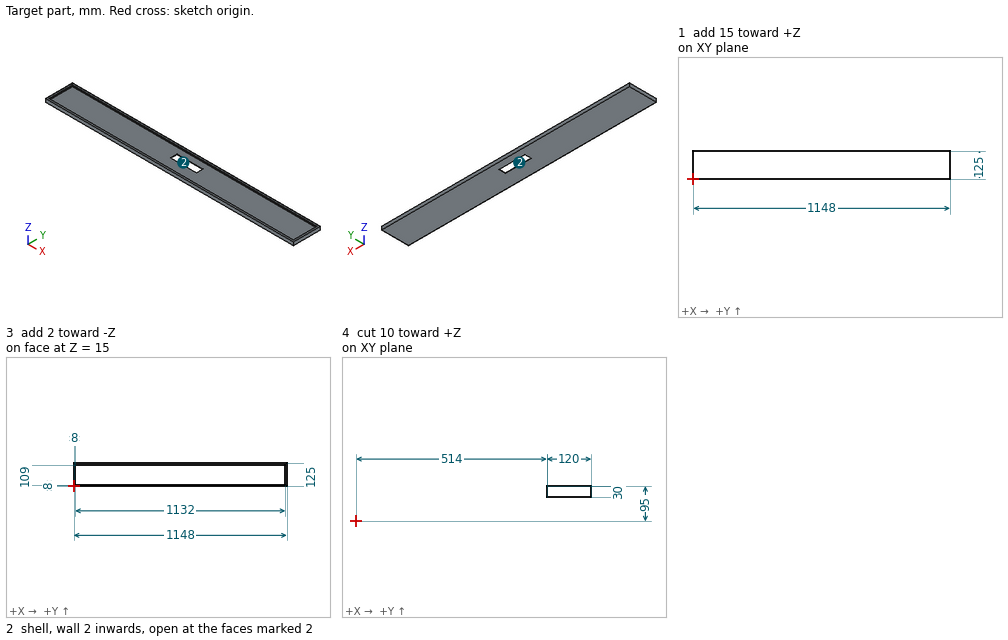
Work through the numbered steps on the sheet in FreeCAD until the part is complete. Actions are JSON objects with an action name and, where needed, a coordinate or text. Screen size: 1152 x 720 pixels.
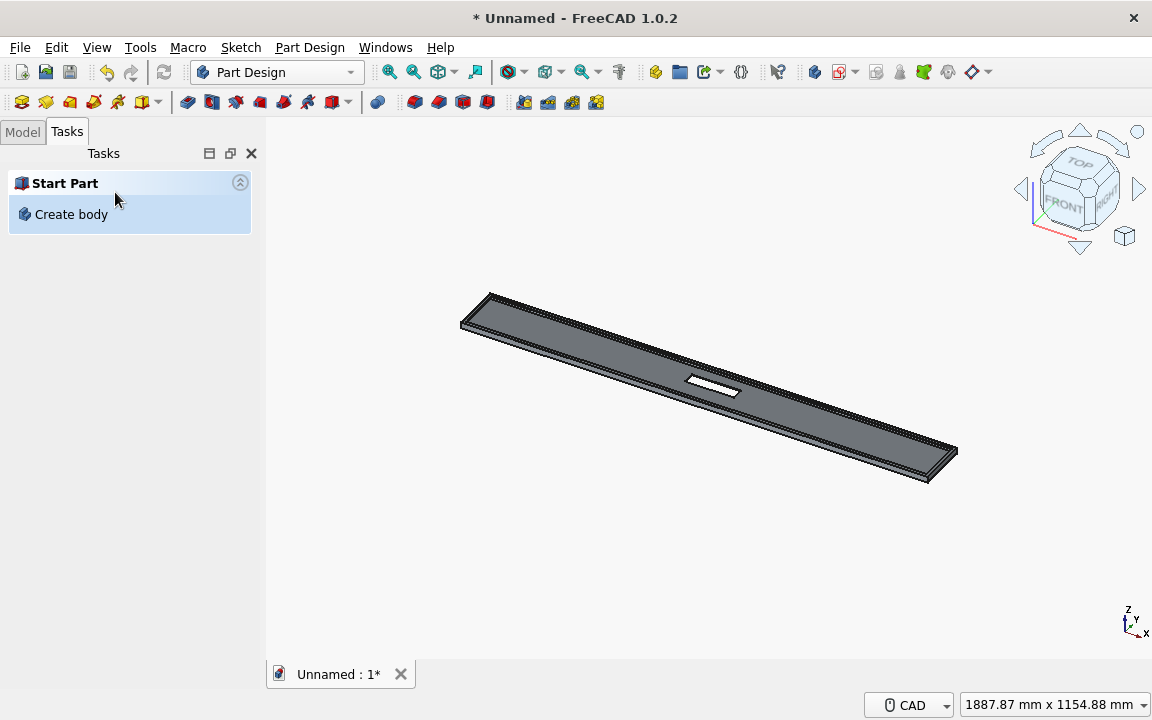
{"action": "key", "text": "0"}